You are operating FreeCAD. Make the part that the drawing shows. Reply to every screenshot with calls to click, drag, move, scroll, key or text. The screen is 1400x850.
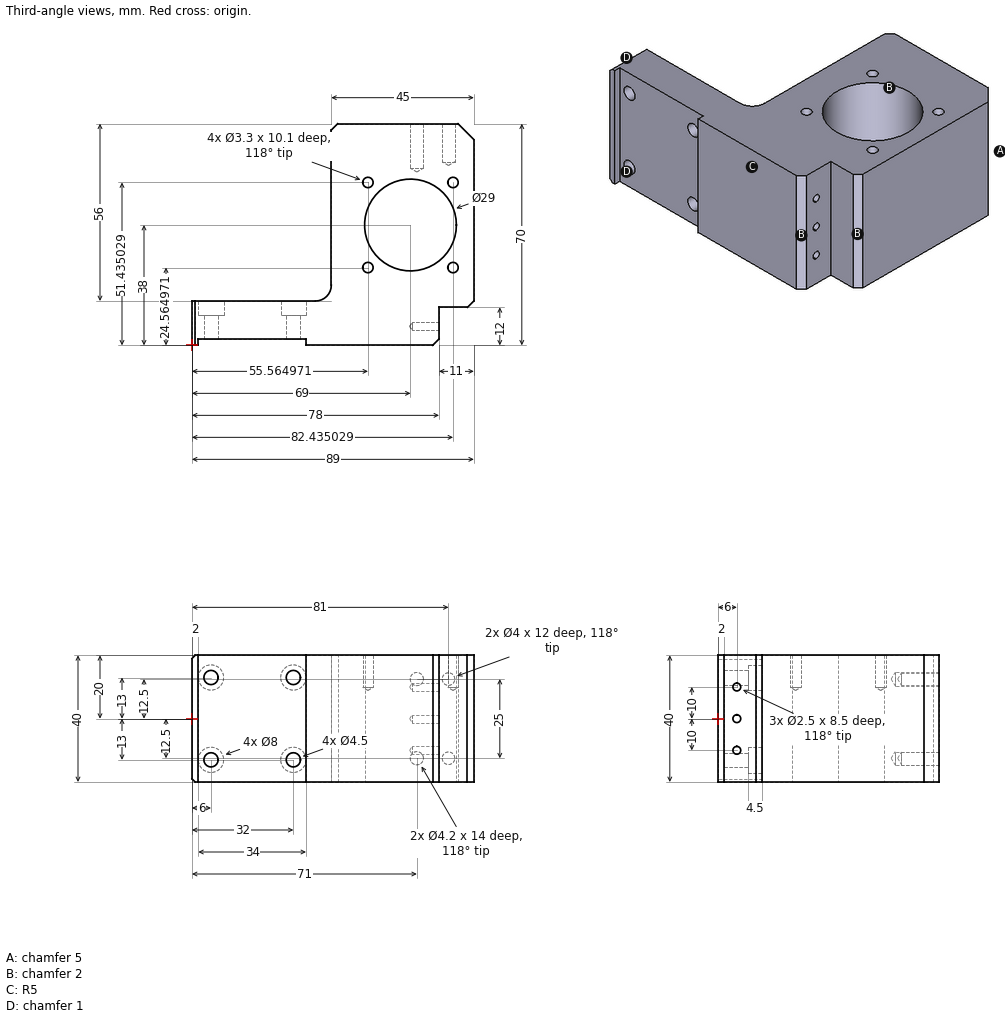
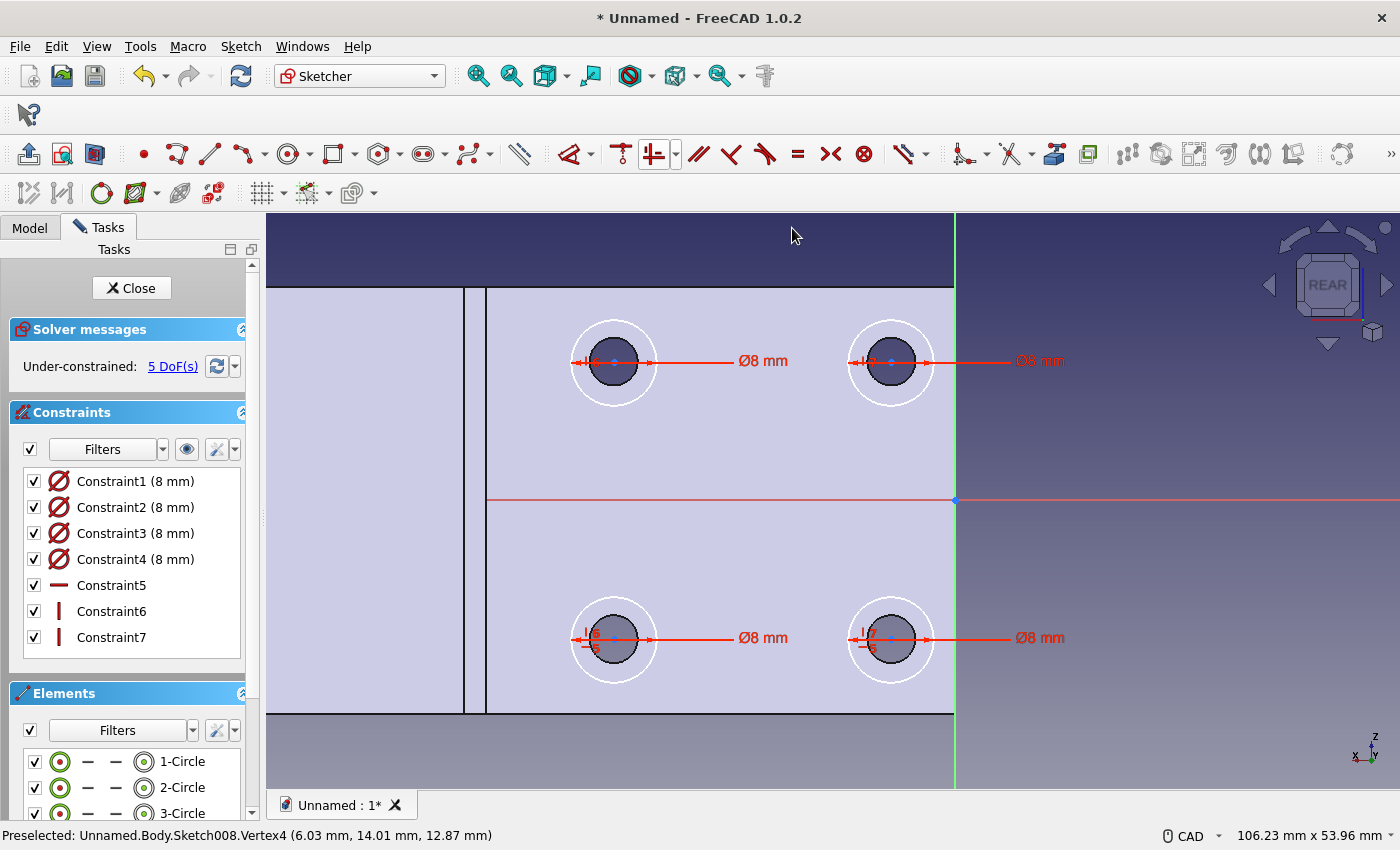
click(614, 363)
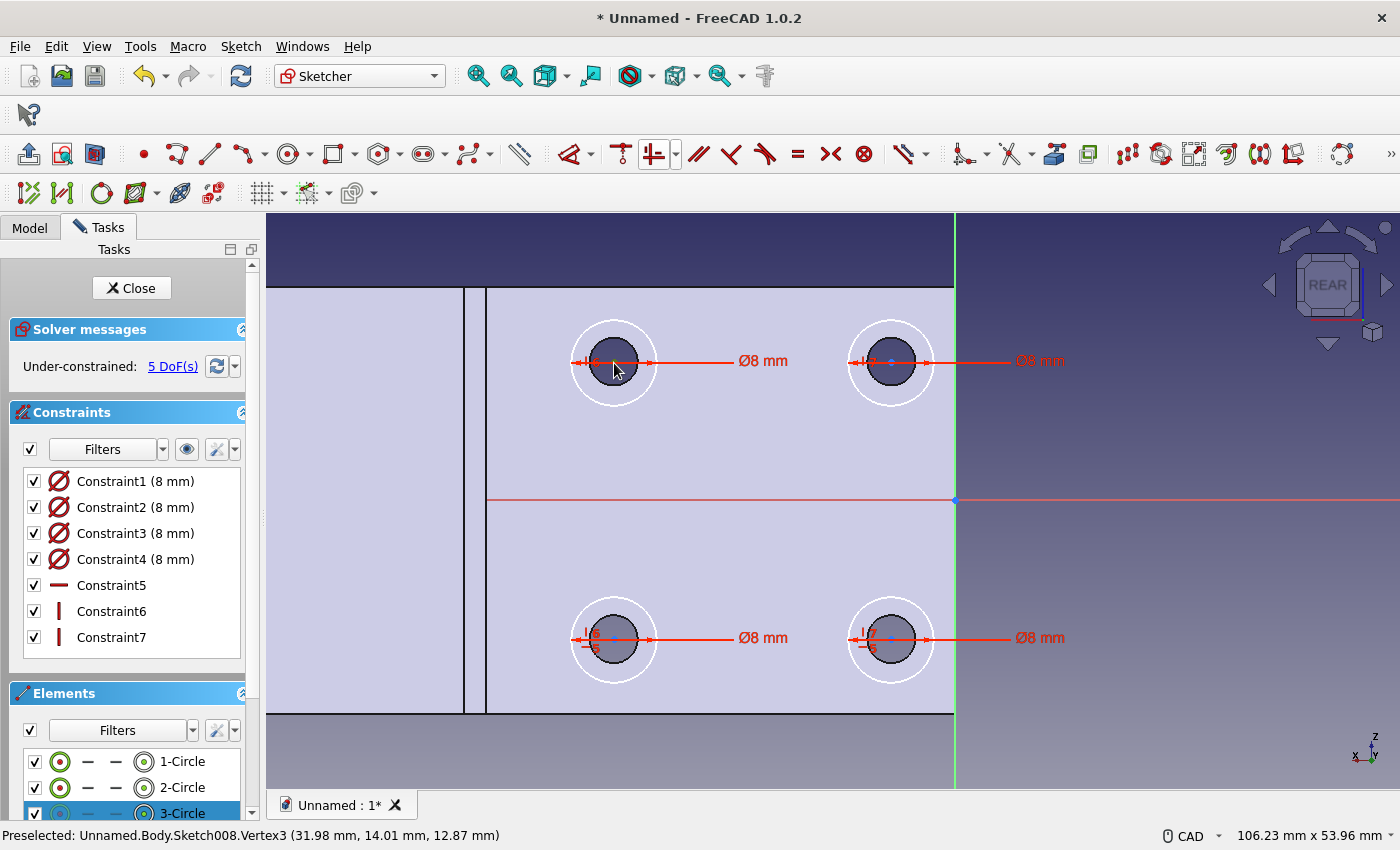
click(891, 363)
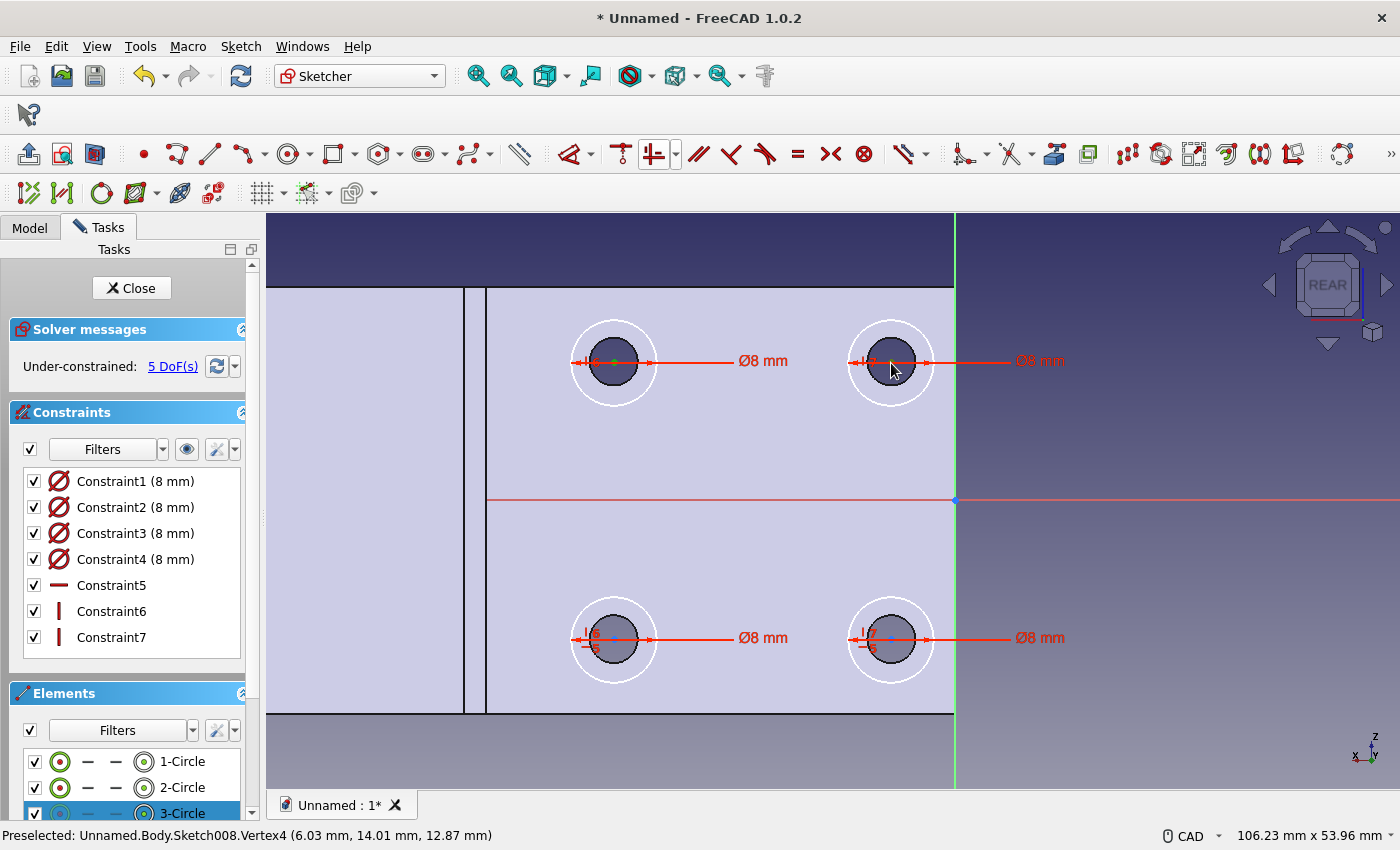
key(h)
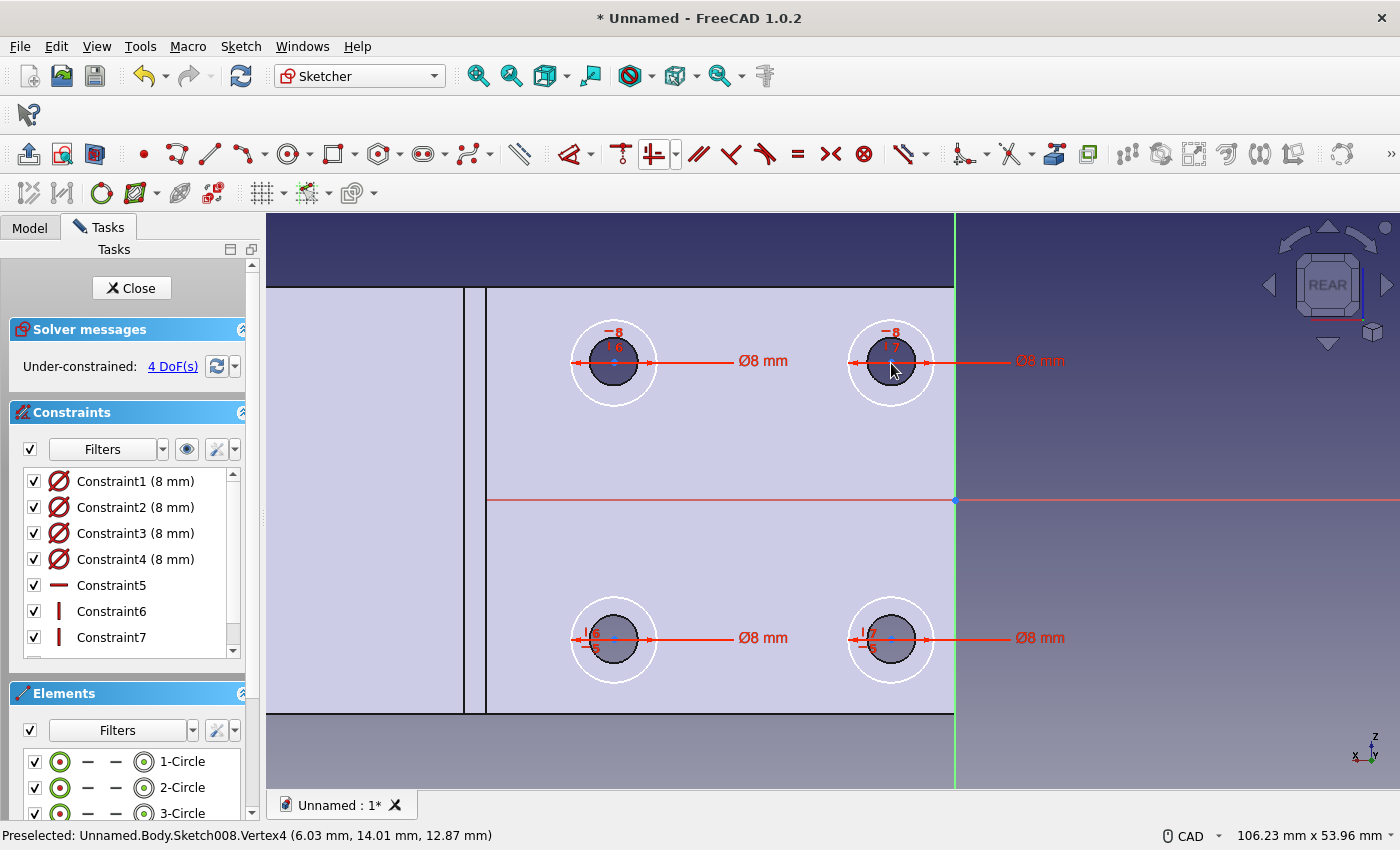
click(568, 154)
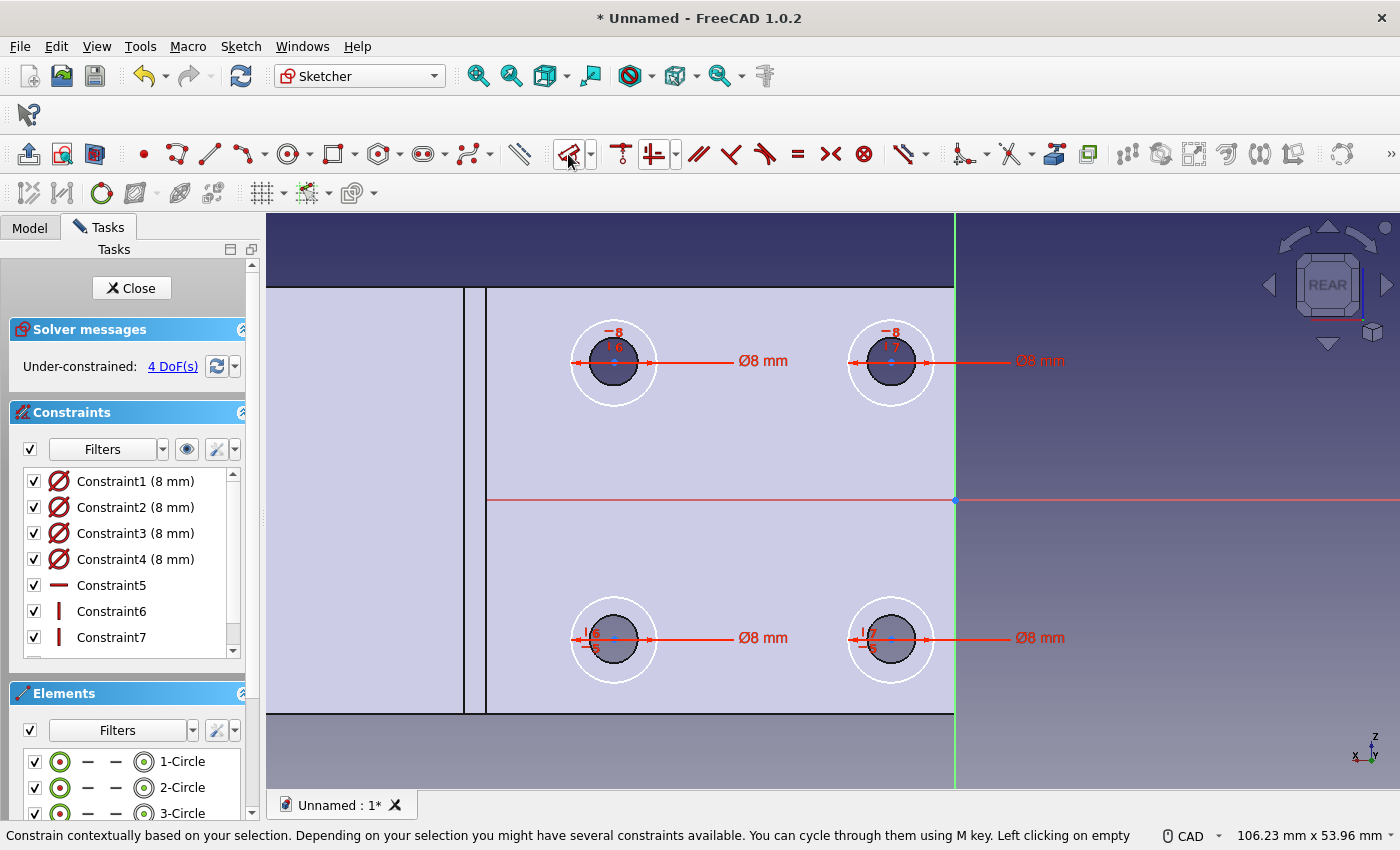
click(891, 640)
click(938, 674)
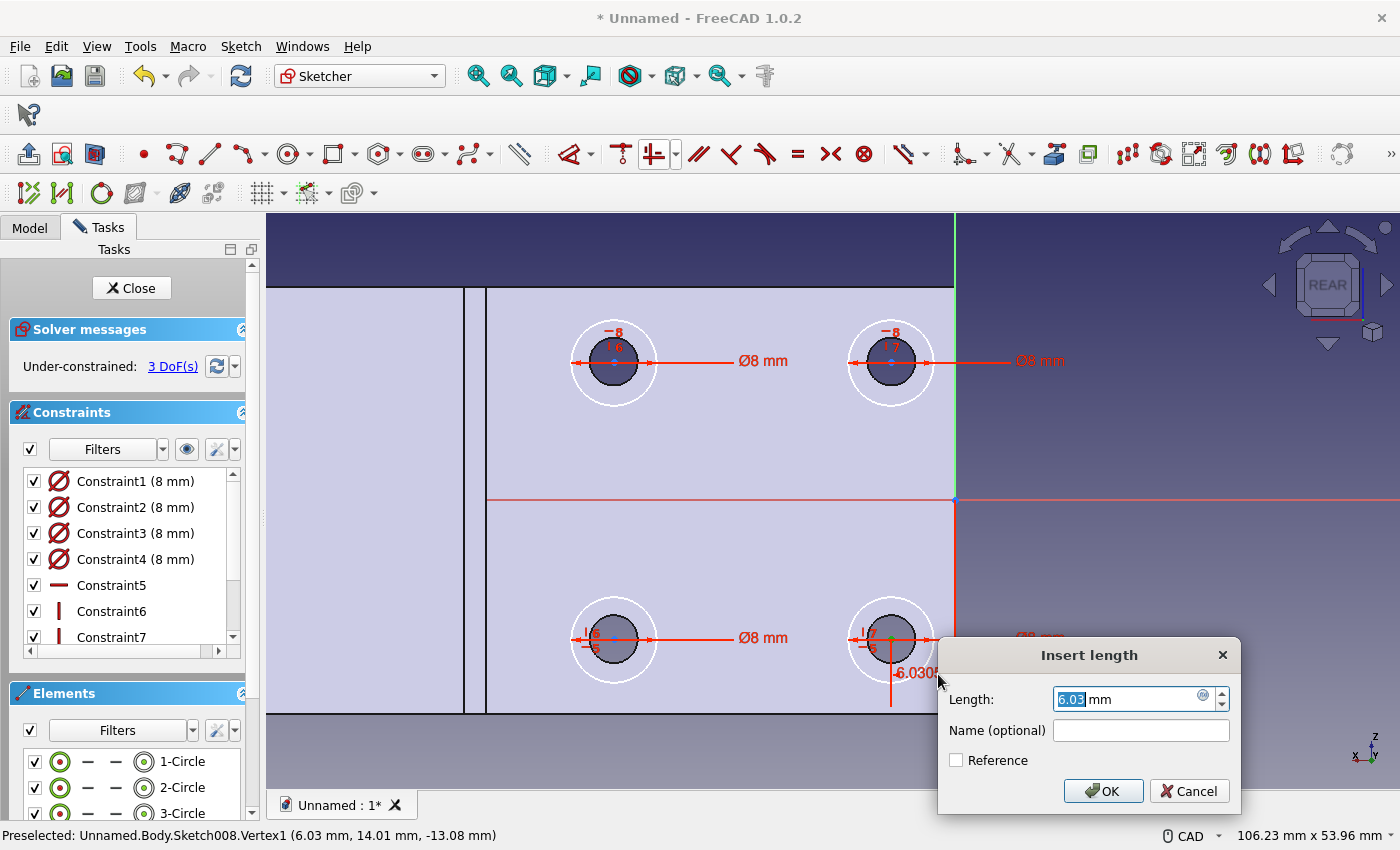
text(6)
key(Return)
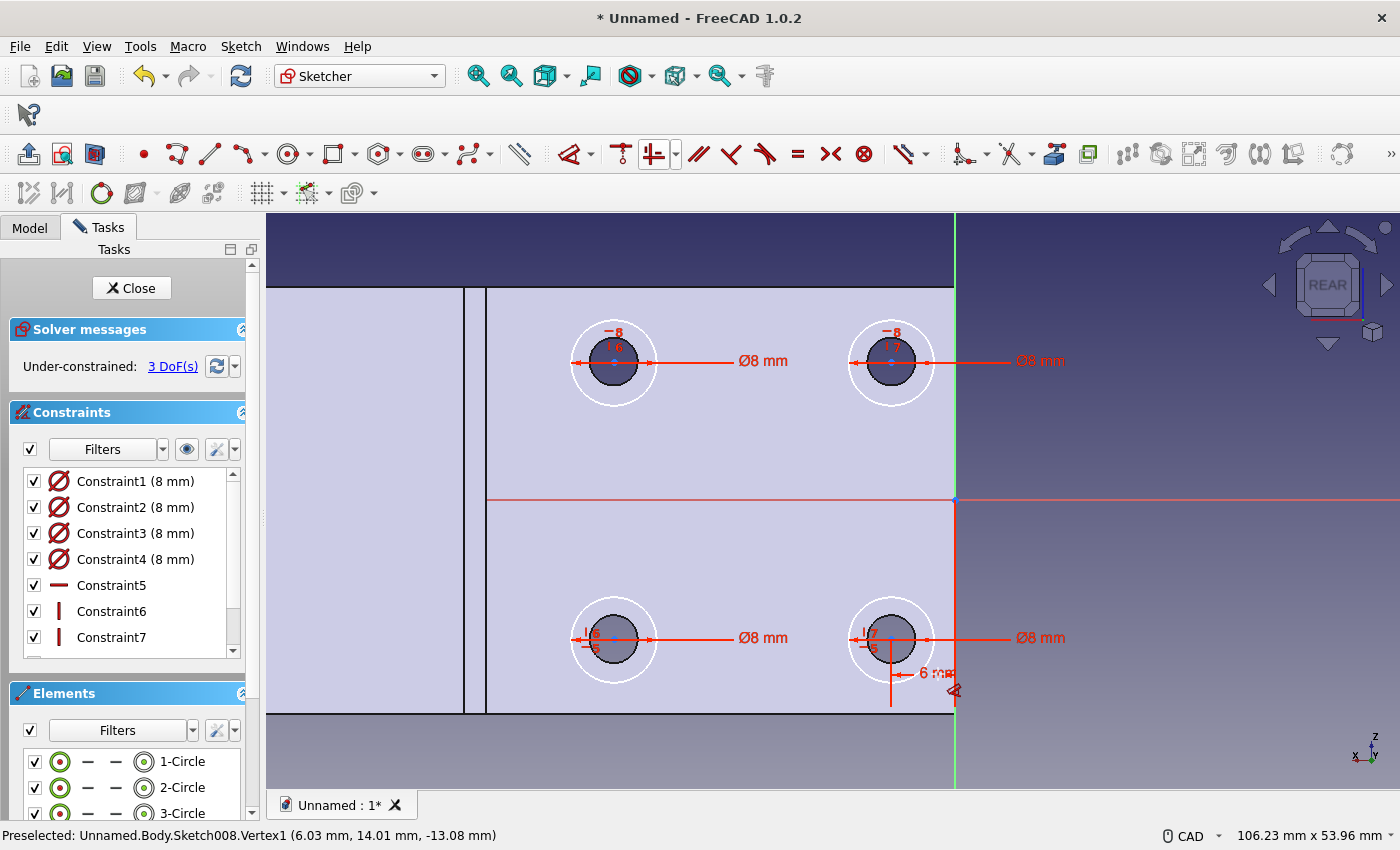
click(891, 640)
click(989, 570)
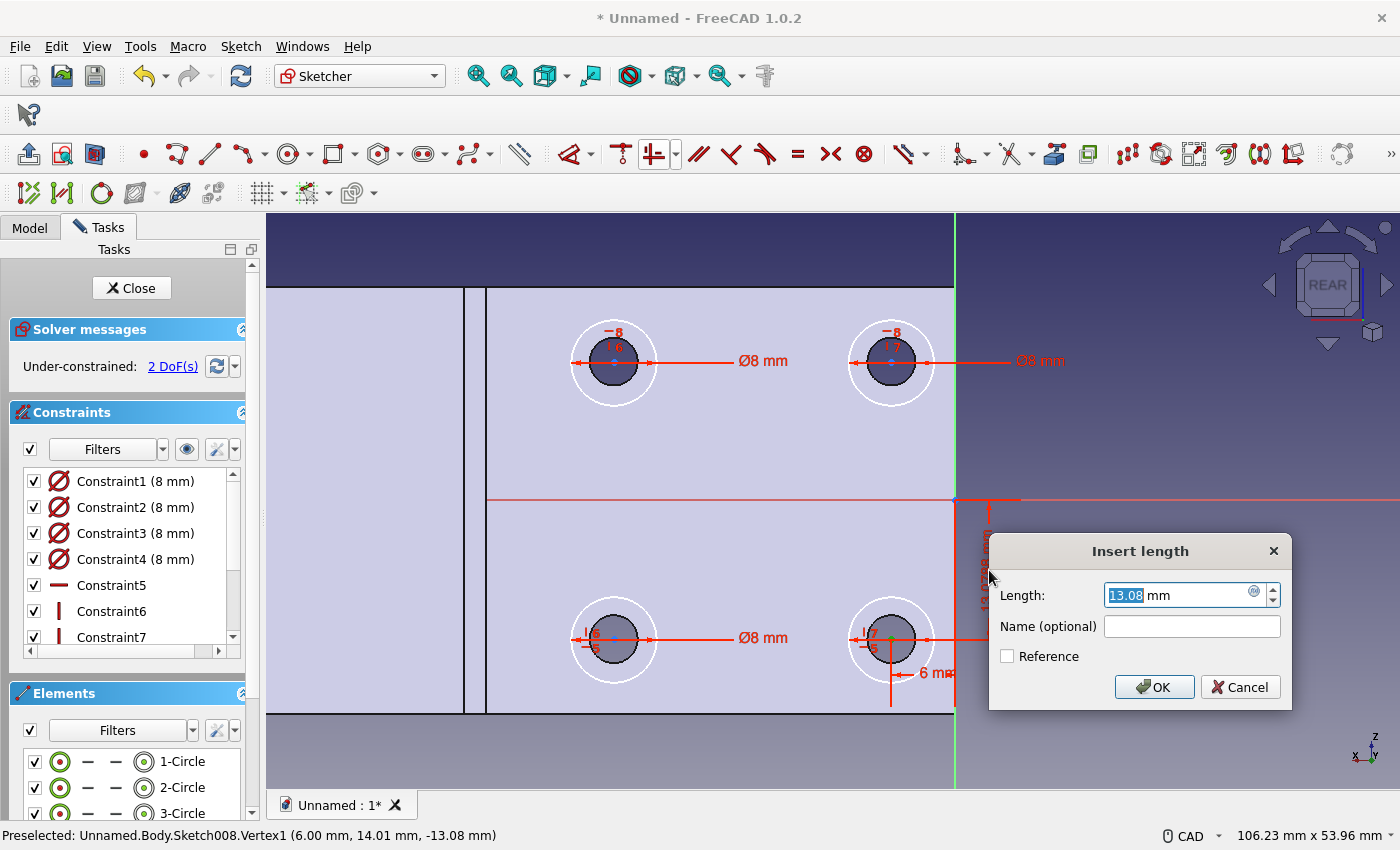
text(13)
key(Return)